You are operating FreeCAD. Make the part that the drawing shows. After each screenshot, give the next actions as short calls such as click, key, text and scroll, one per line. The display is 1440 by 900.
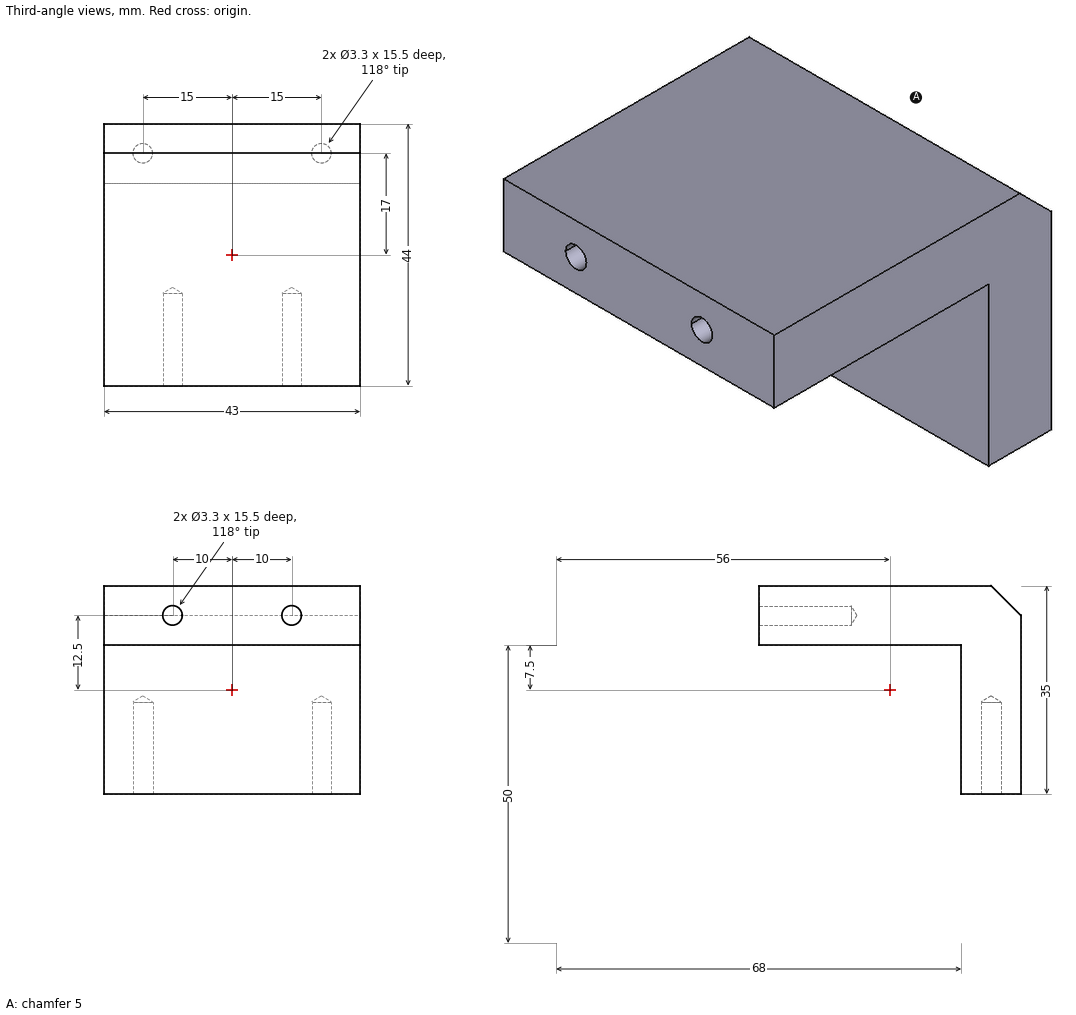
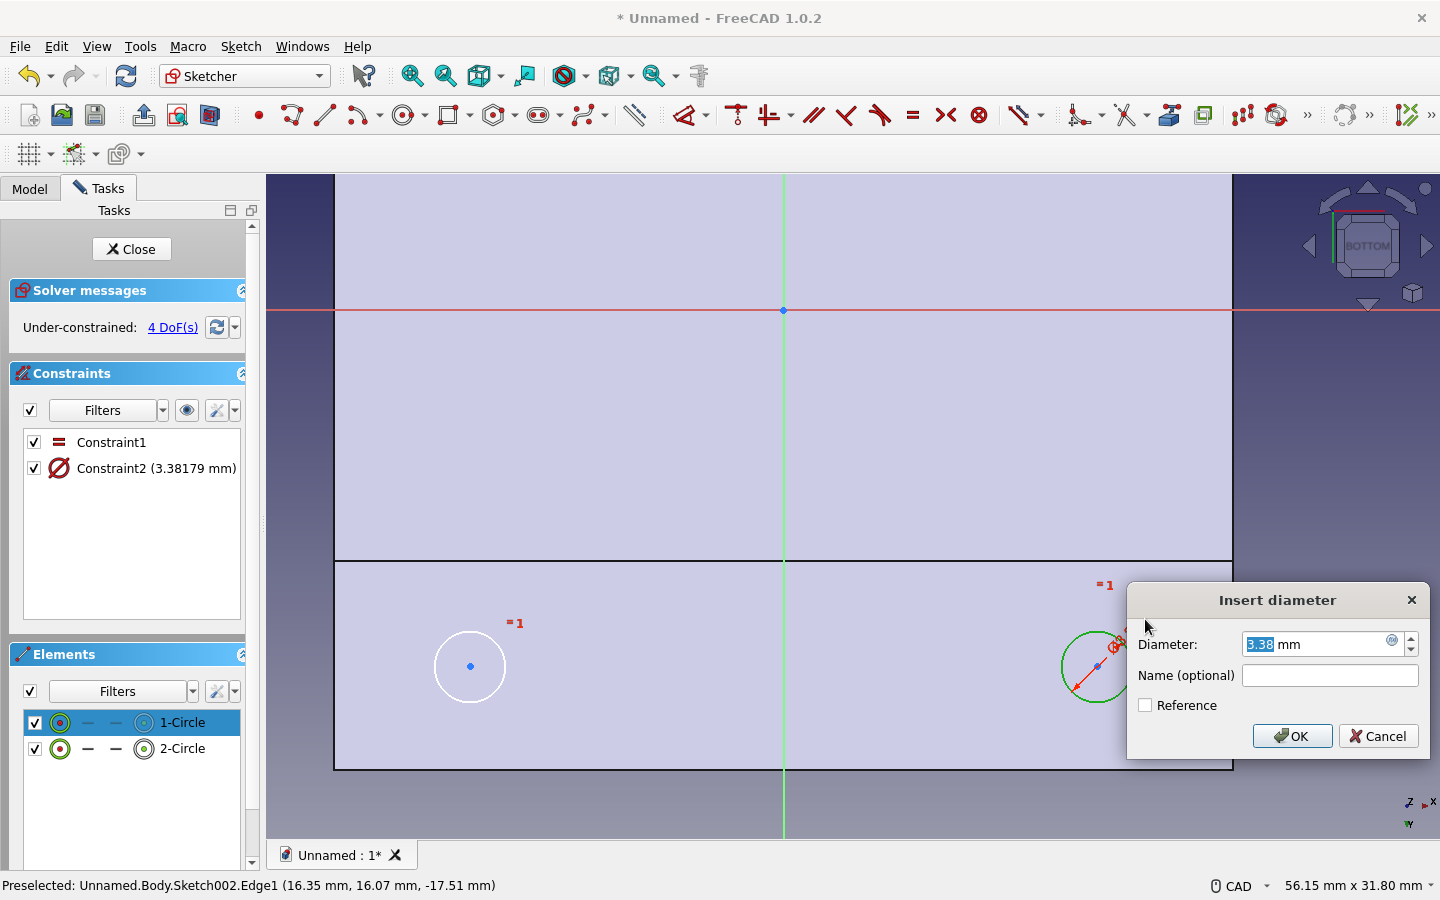
text(3.3)
key(Return)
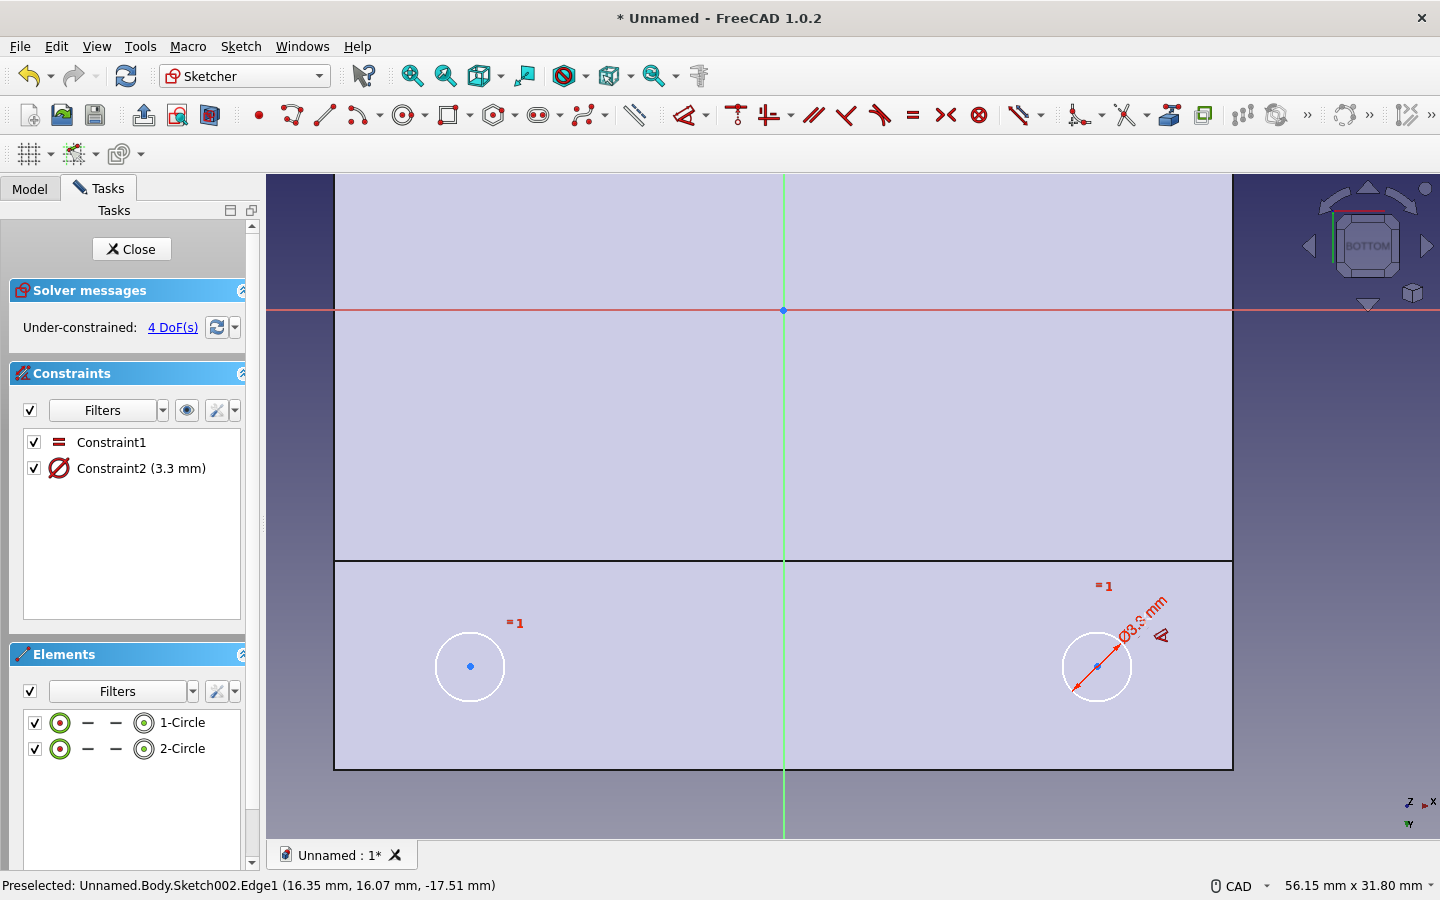
click(1097, 667)
click(940, 276)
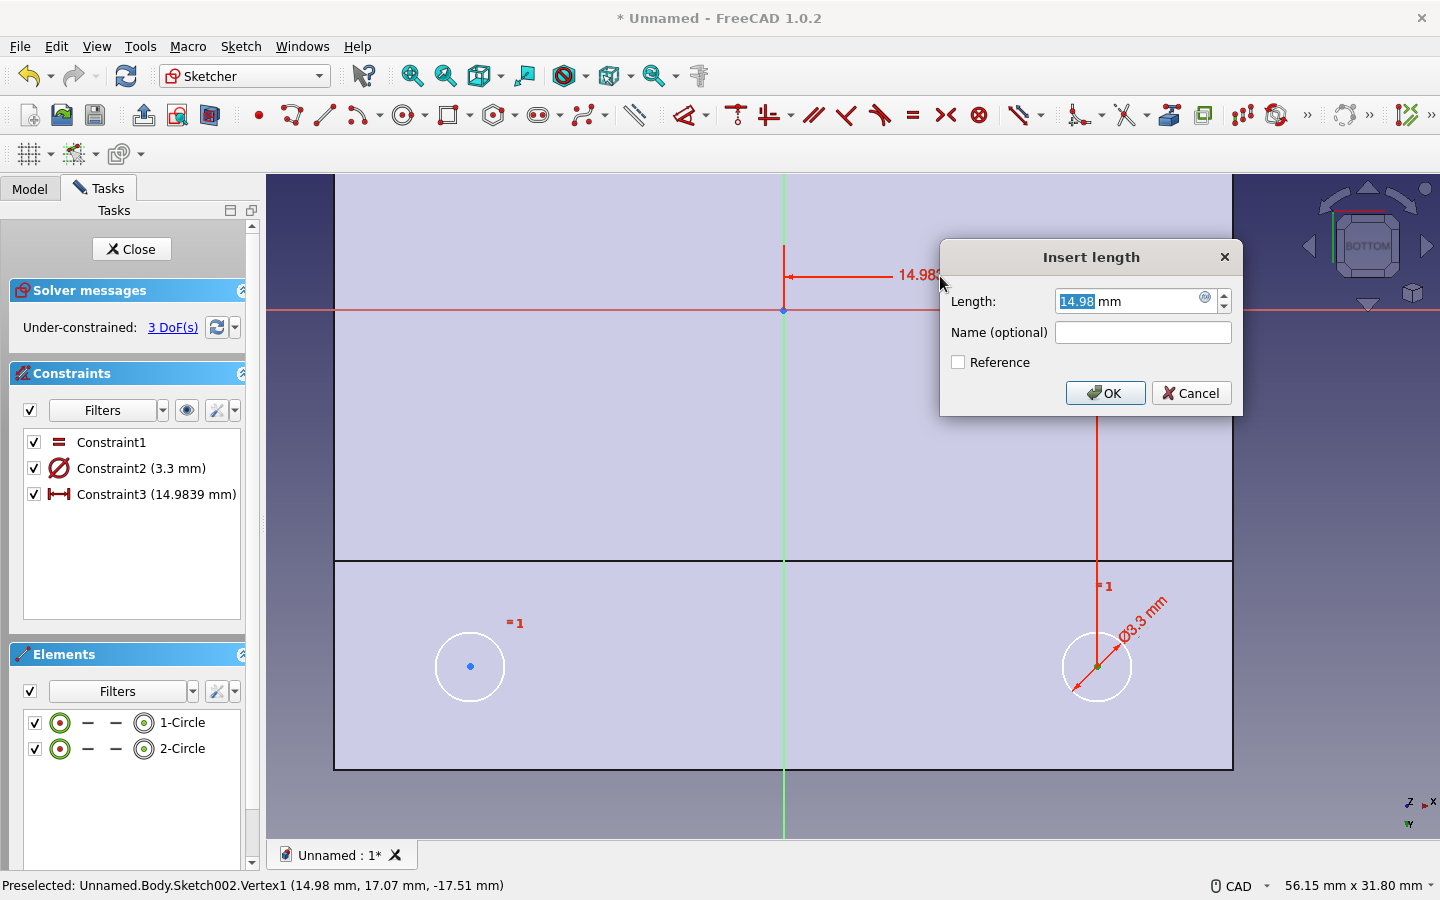
text(15)
key(Return)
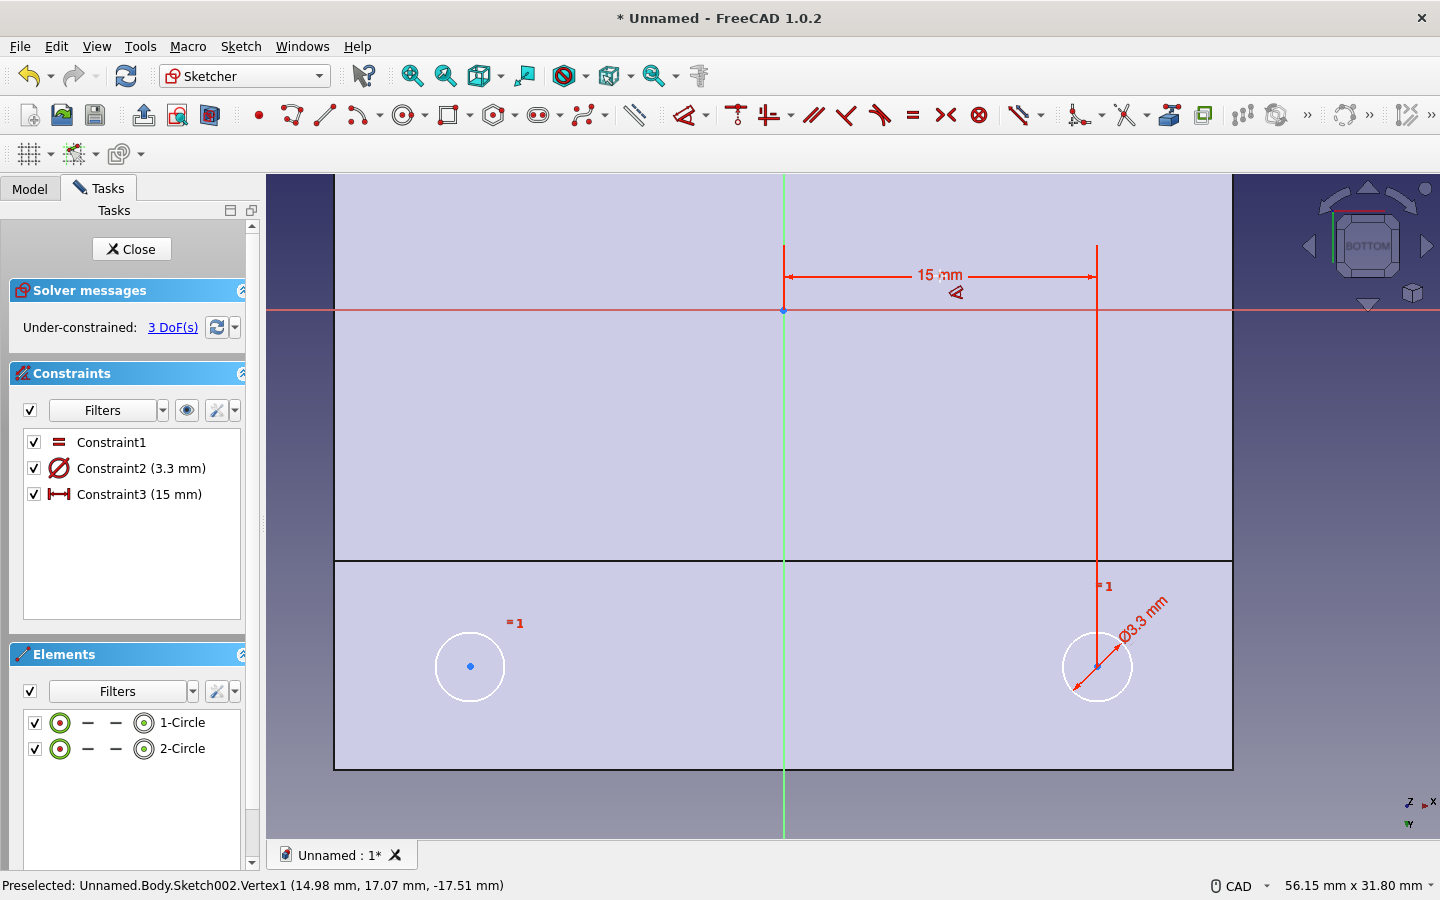
click(1097, 667)
click(1131, 489)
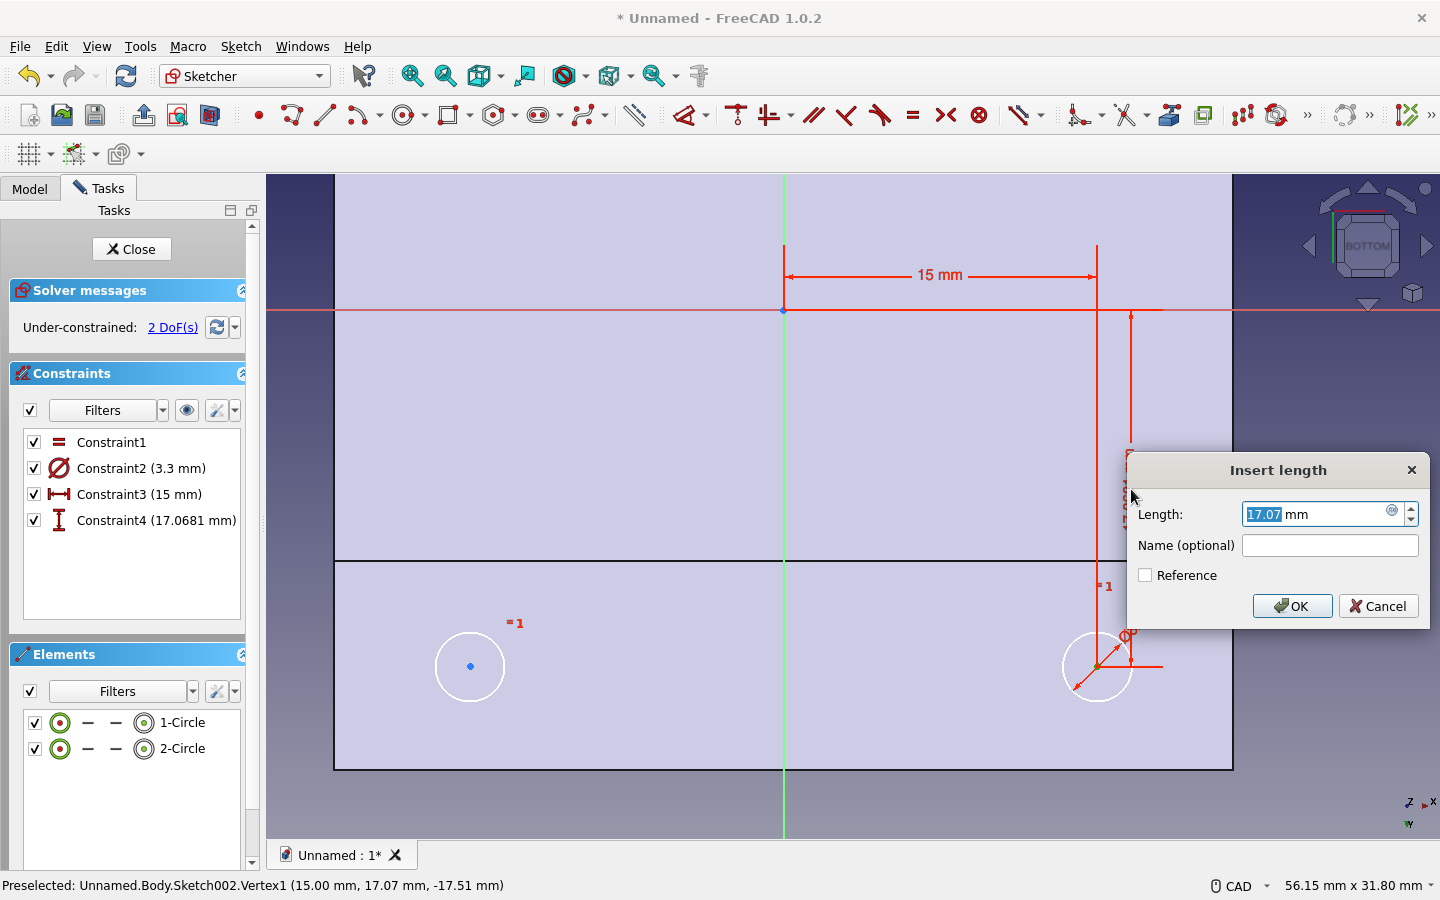
text(17)
key(Return)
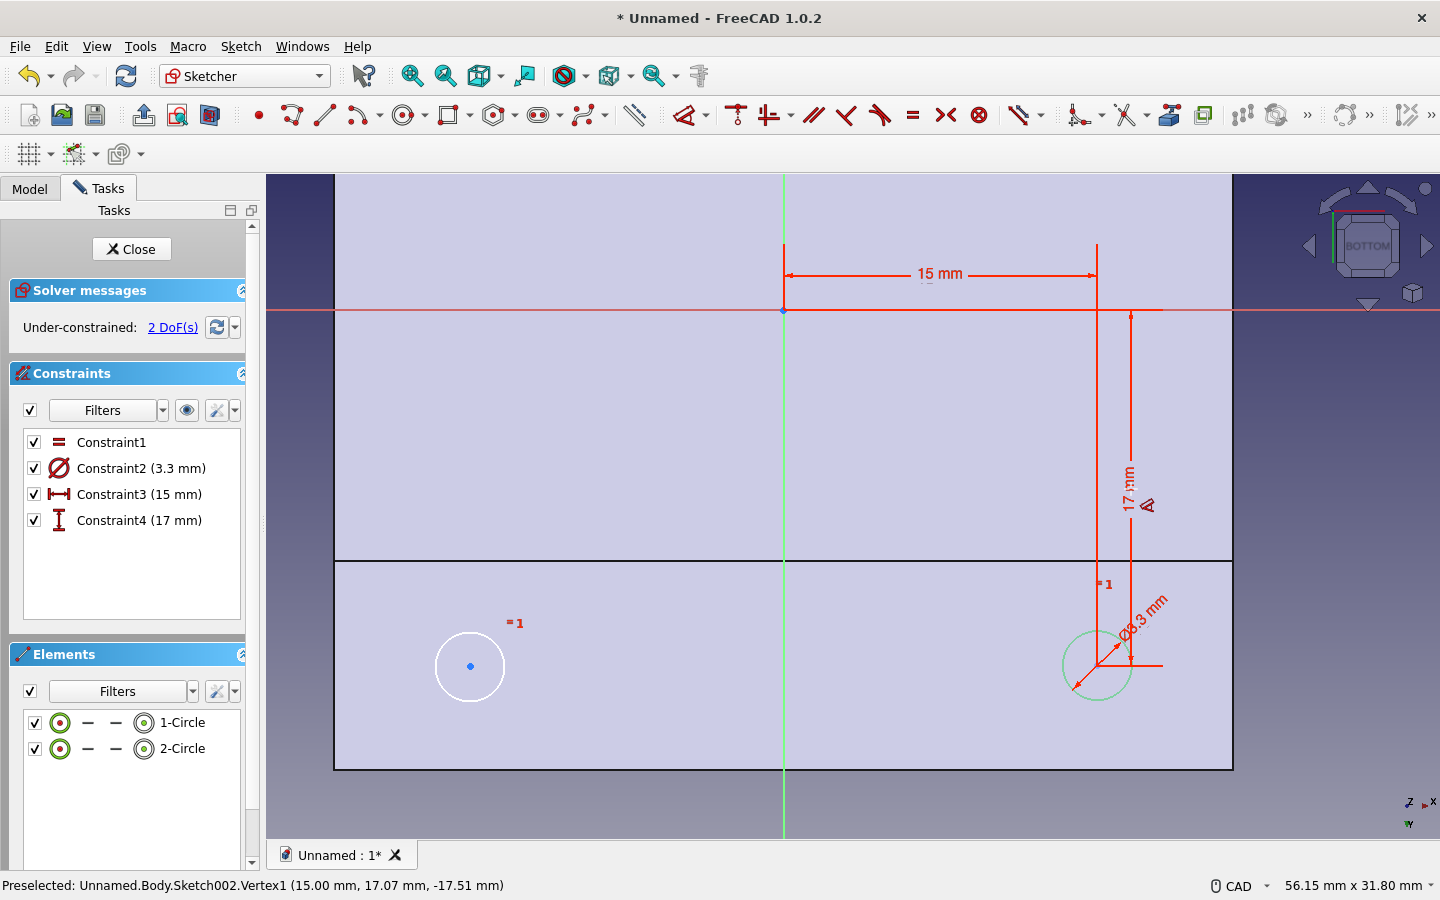
click(470, 667)
click(627, 276)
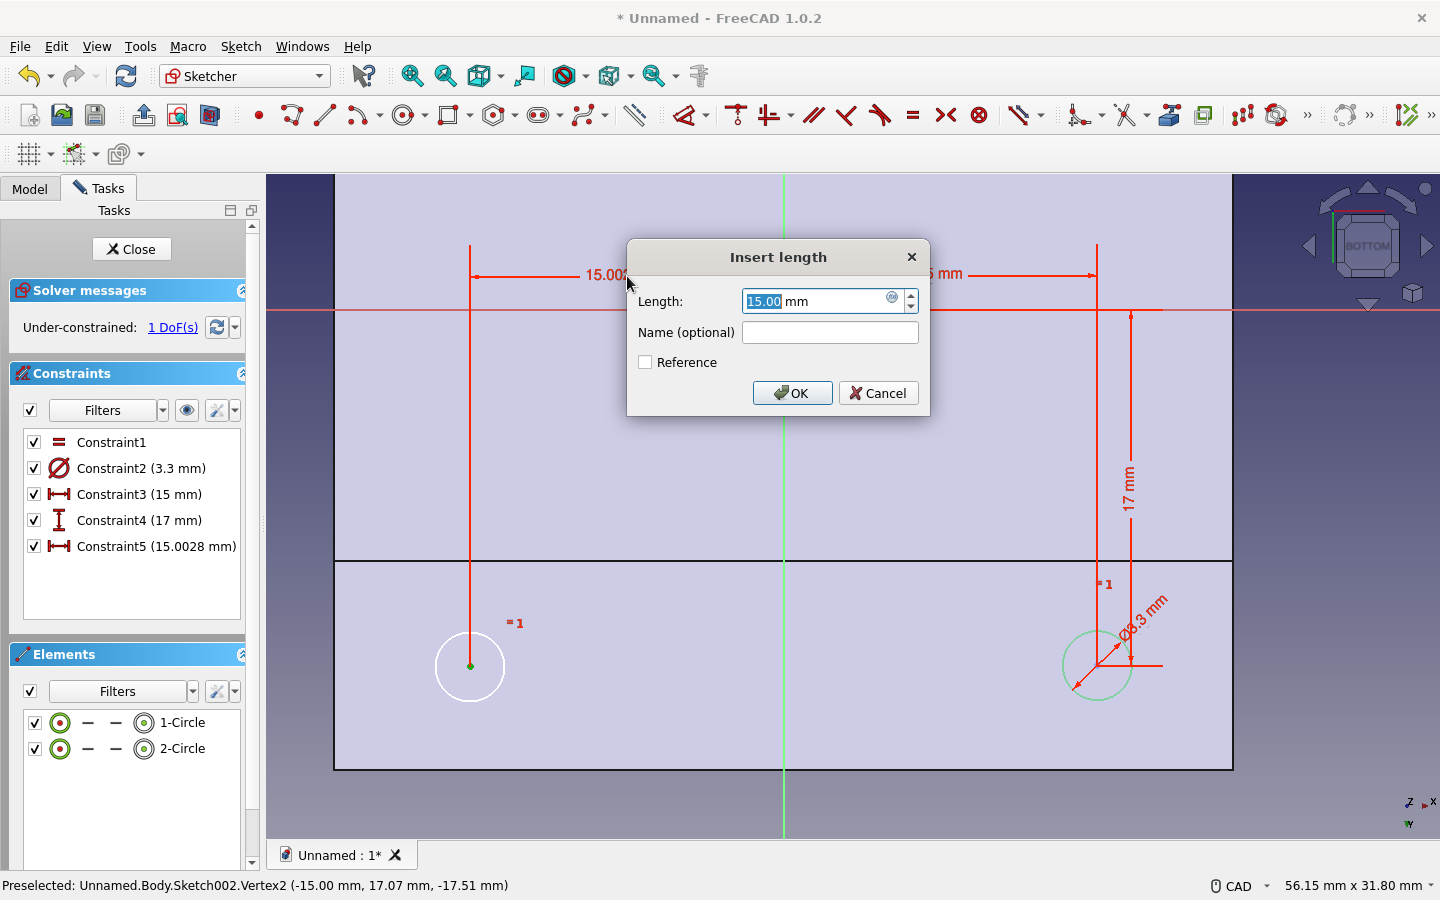
text(15)
key(Return)